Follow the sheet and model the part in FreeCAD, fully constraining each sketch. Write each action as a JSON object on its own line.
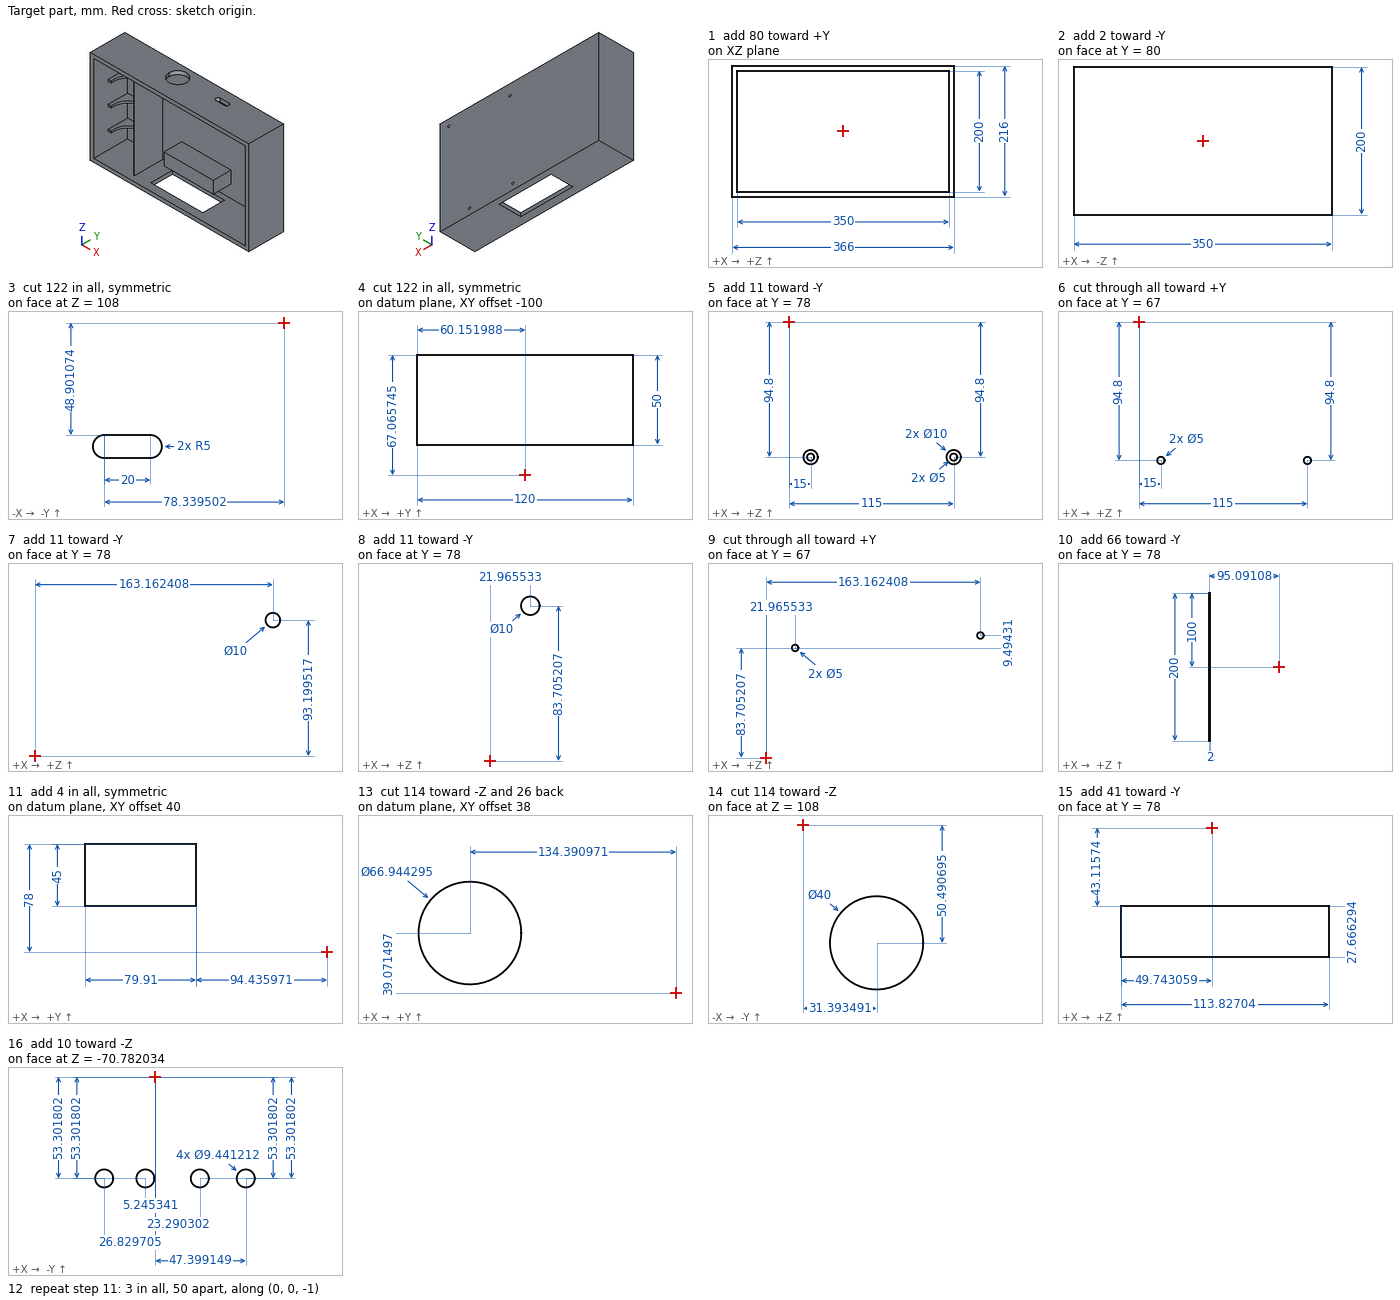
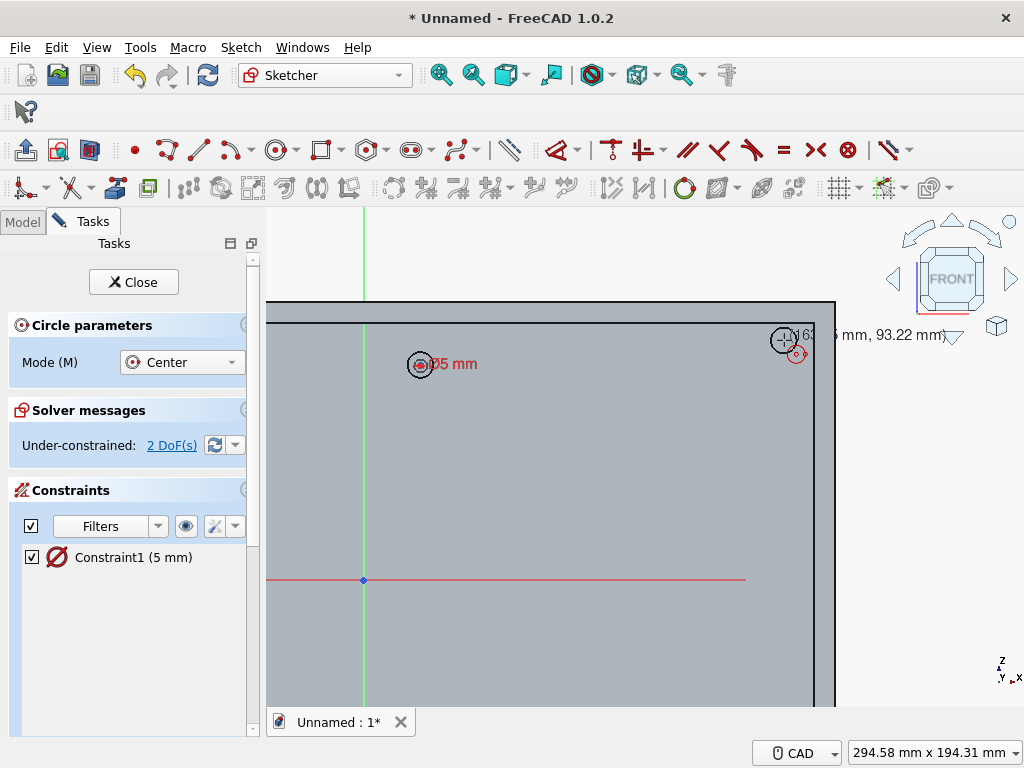
{"action": "left_click", "coordinate": [784, 340]}
{"action": "mouse_move", "coordinate": [788, 336]}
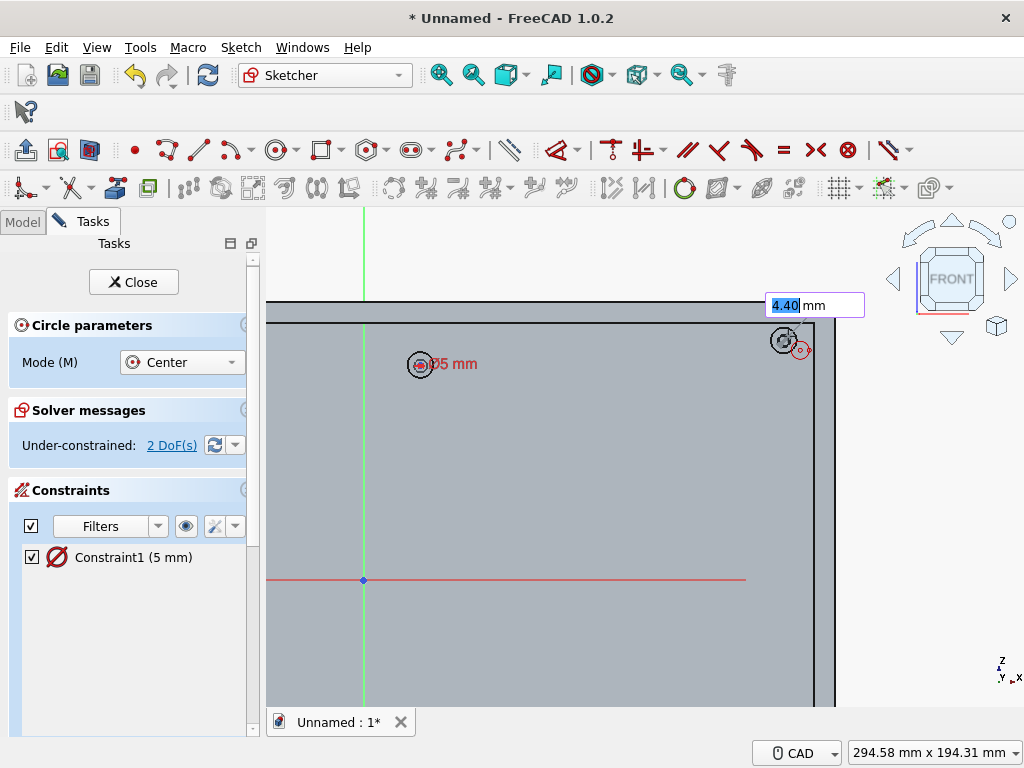
{"action": "type", "text": "5"}
{"action": "key", "text": "Return"}
{"action": "key", "text": "Escape"}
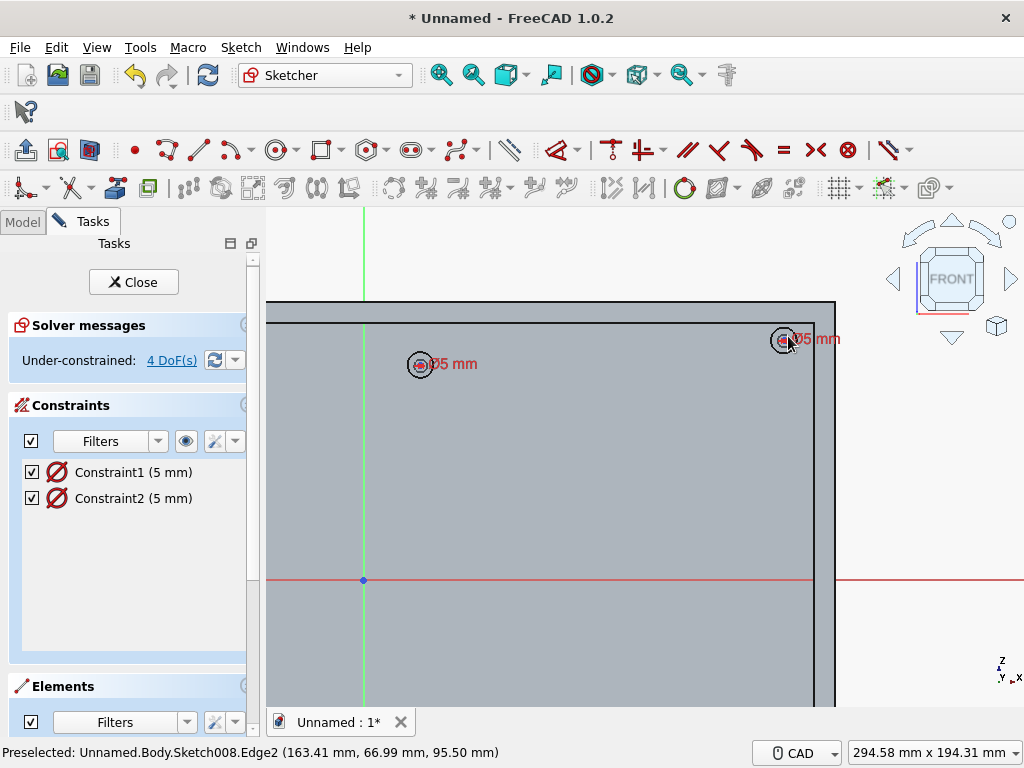
{"action": "left_click", "coordinate": [556, 150]}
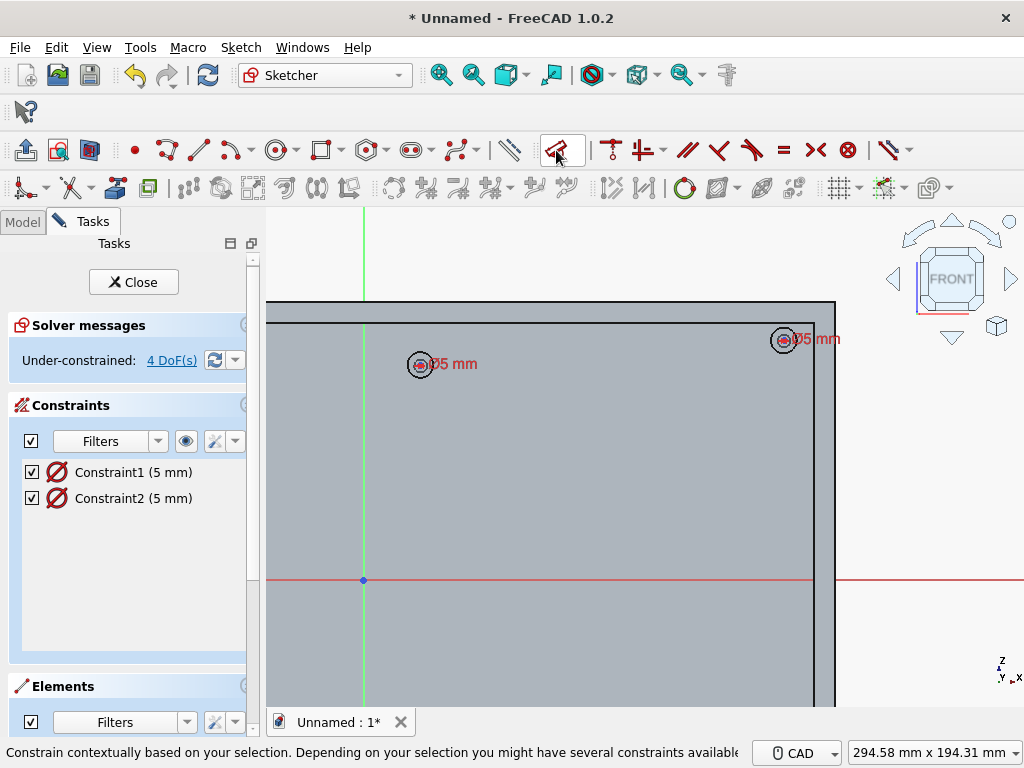
{"action": "scroll", "coordinate": [421, 366], "scroll_direction": "up", "scroll_amount": 3}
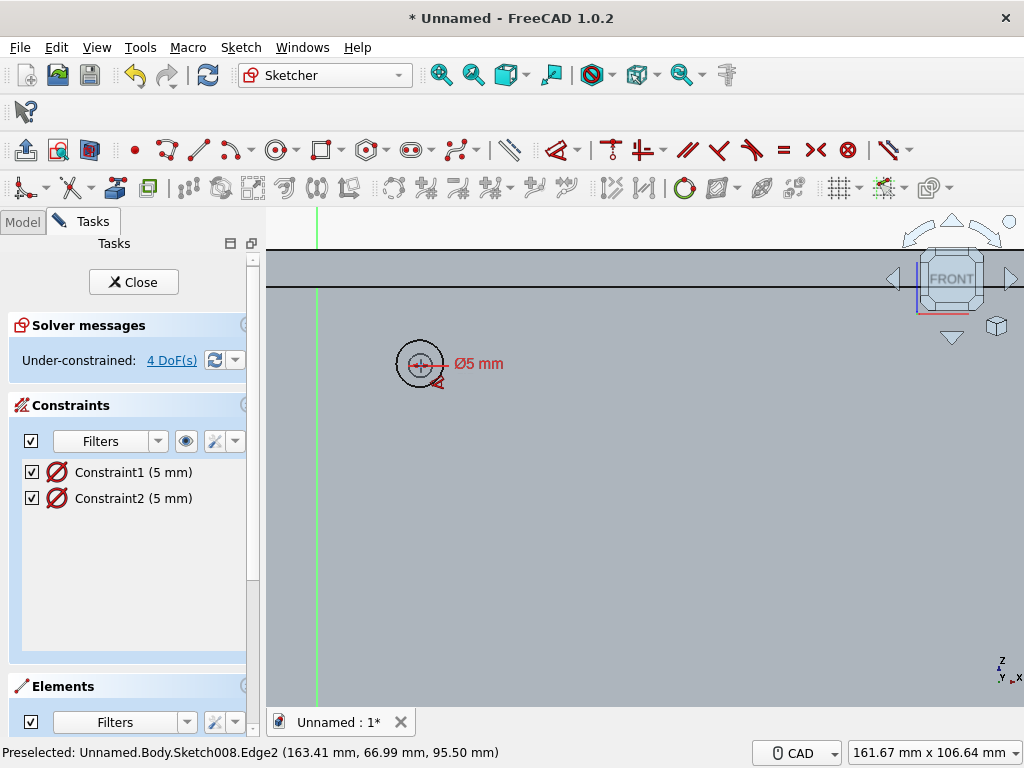
{"action": "left_click", "coordinate": [420, 366]}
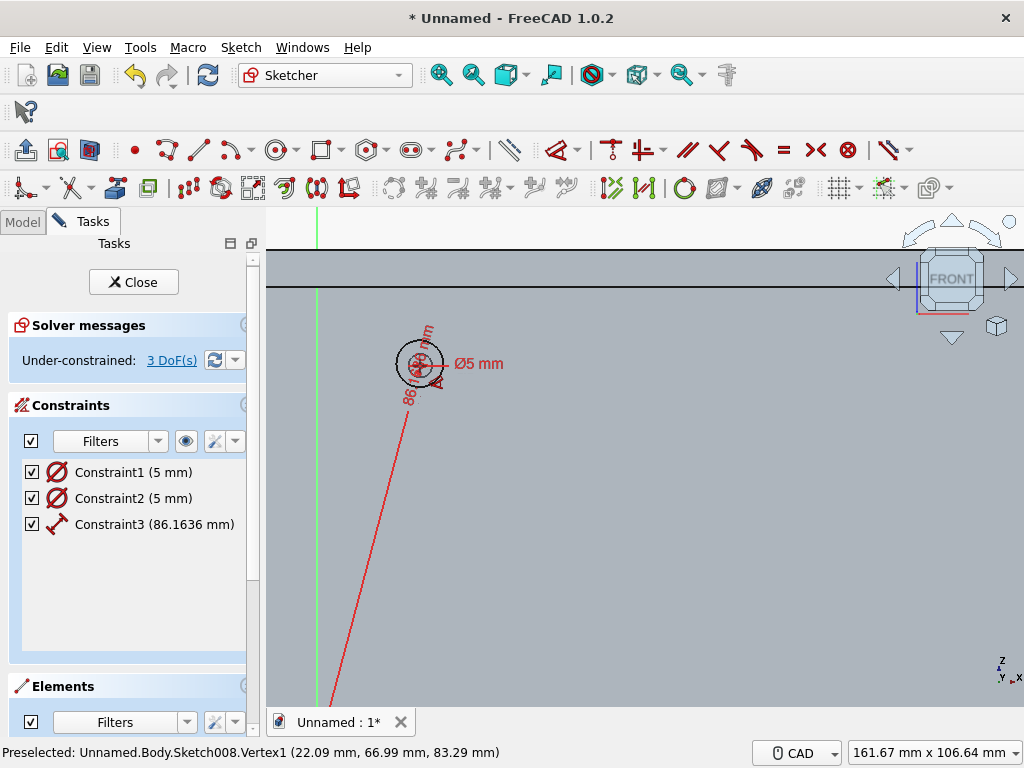
{"action": "scroll", "coordinate": [420, 366], "scroll_direction": "down", "scroll_amount": 3}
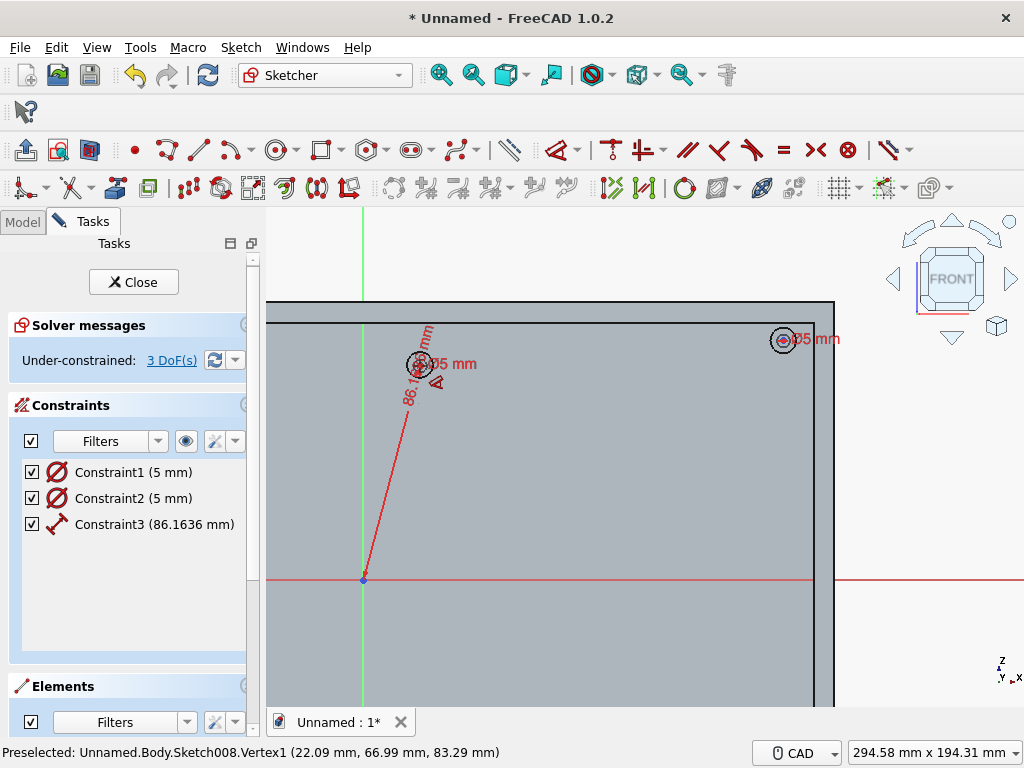
{"action": "scroll", "coordinate": [784, 341], "scroll_direction": "up", "scroll_amount": 3}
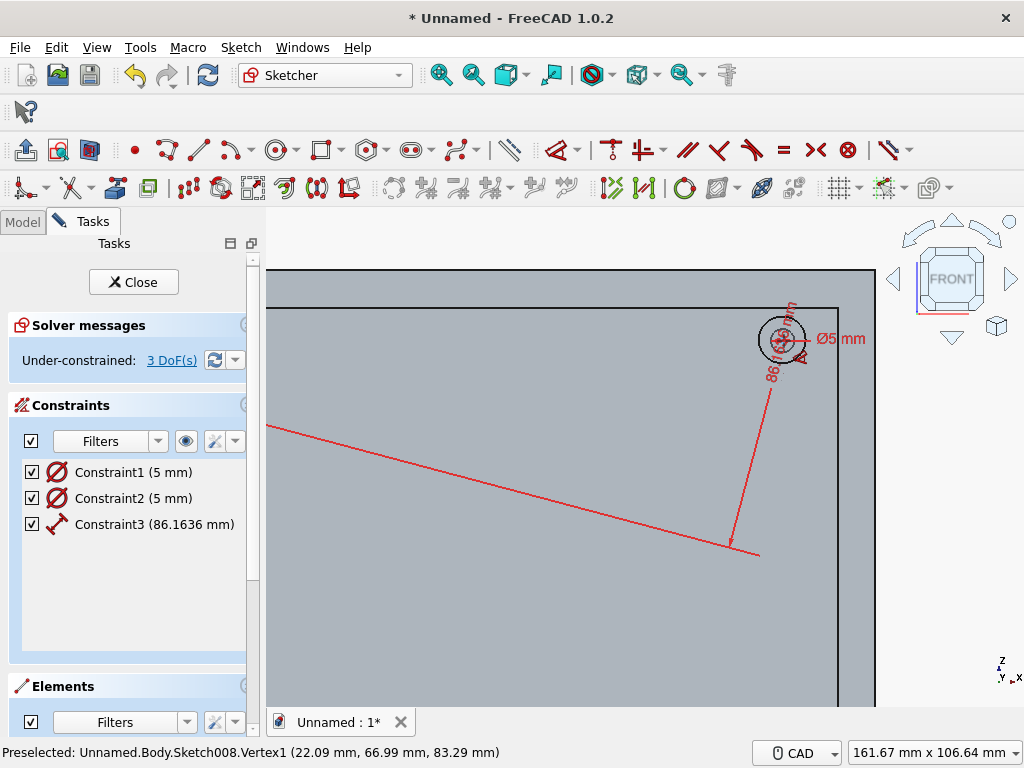
{"action": "left_click", "coordinate": [783, 341]}
{"action": "left_click", "coordinate": [817, 364]}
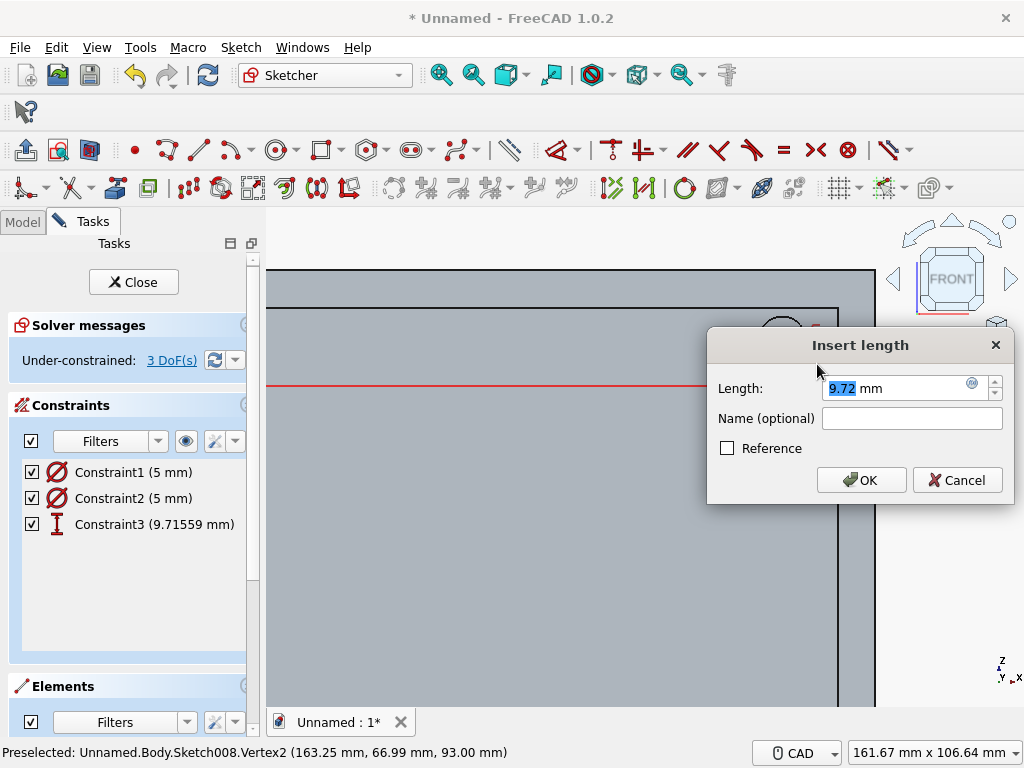
{"action": "type", "text": "9.49431"}
{"action": "key", "text": "Return"}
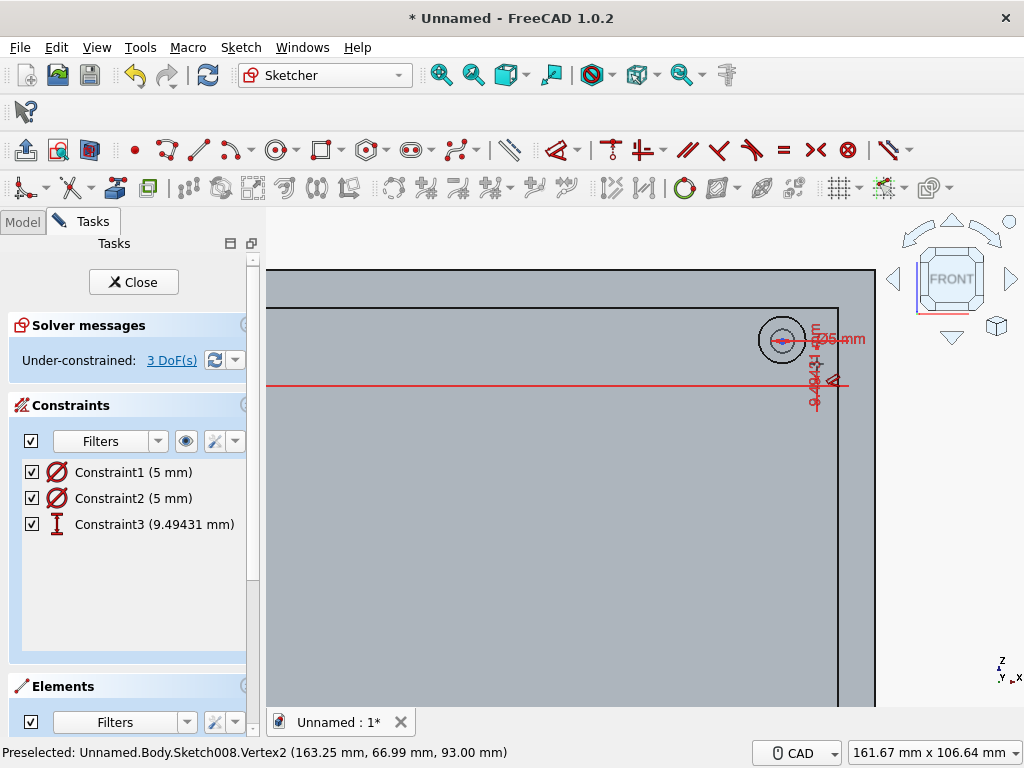
{"action": "scroll", "coordinate": [784, 341], "scroll_direction": "down", "scroll_amount": 3}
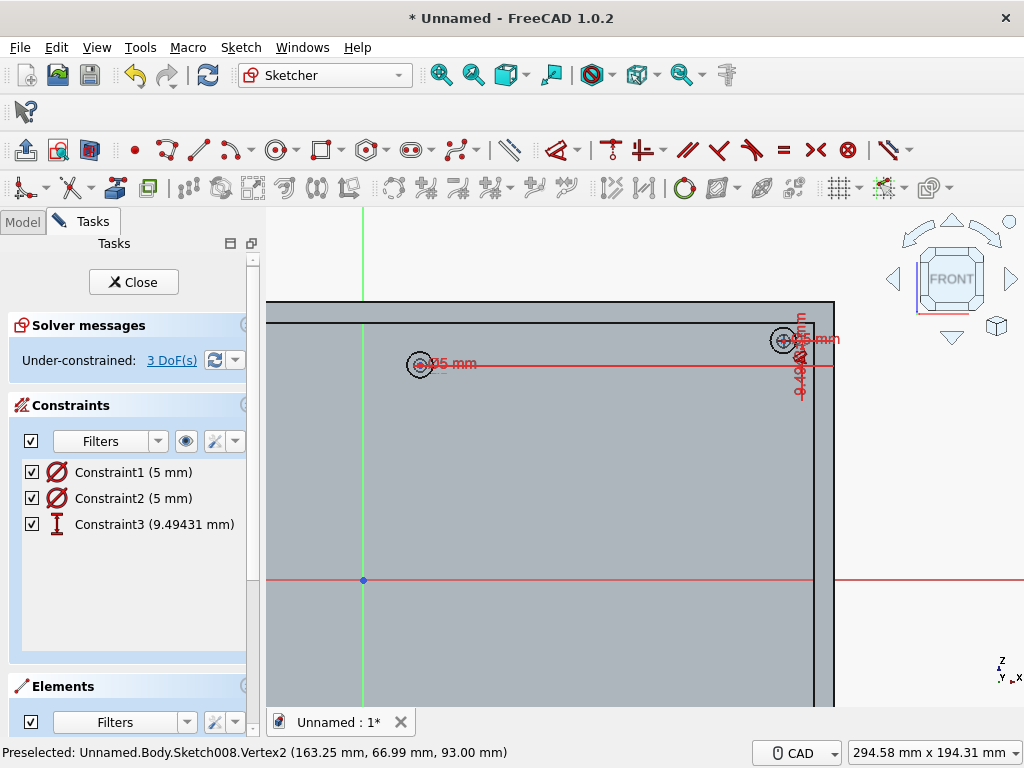
{"action": "left_click", "coordinate": [420, 366]}
{"action": "left_click", "coordinate": [392, 614]}